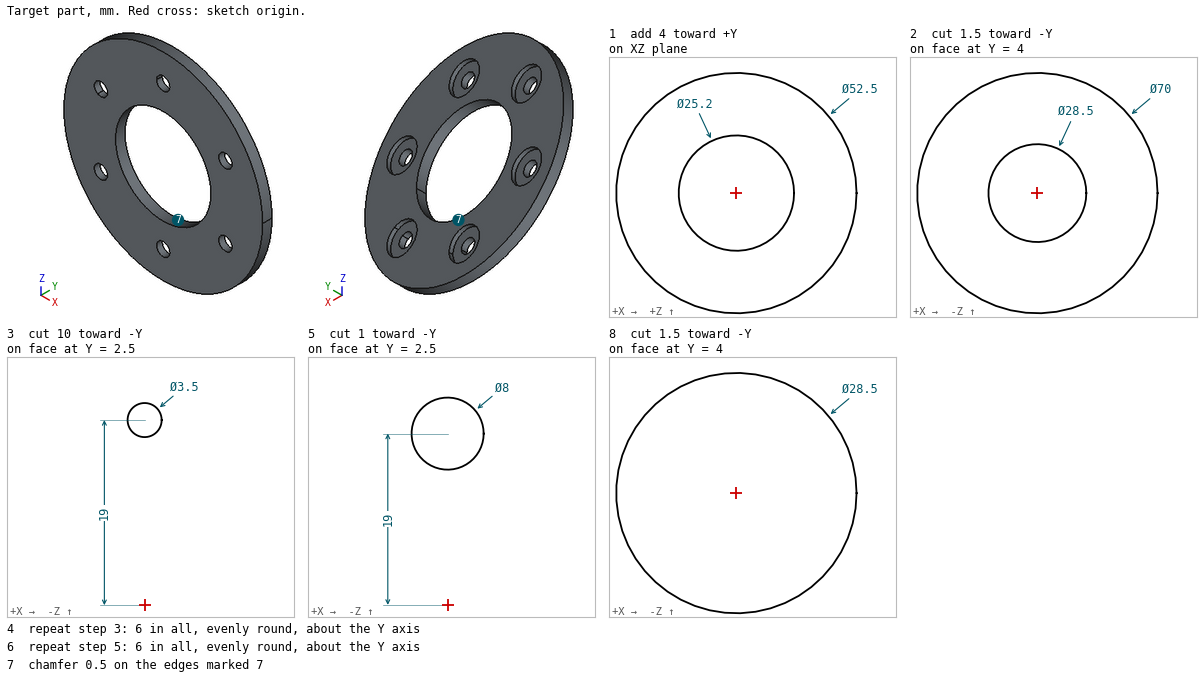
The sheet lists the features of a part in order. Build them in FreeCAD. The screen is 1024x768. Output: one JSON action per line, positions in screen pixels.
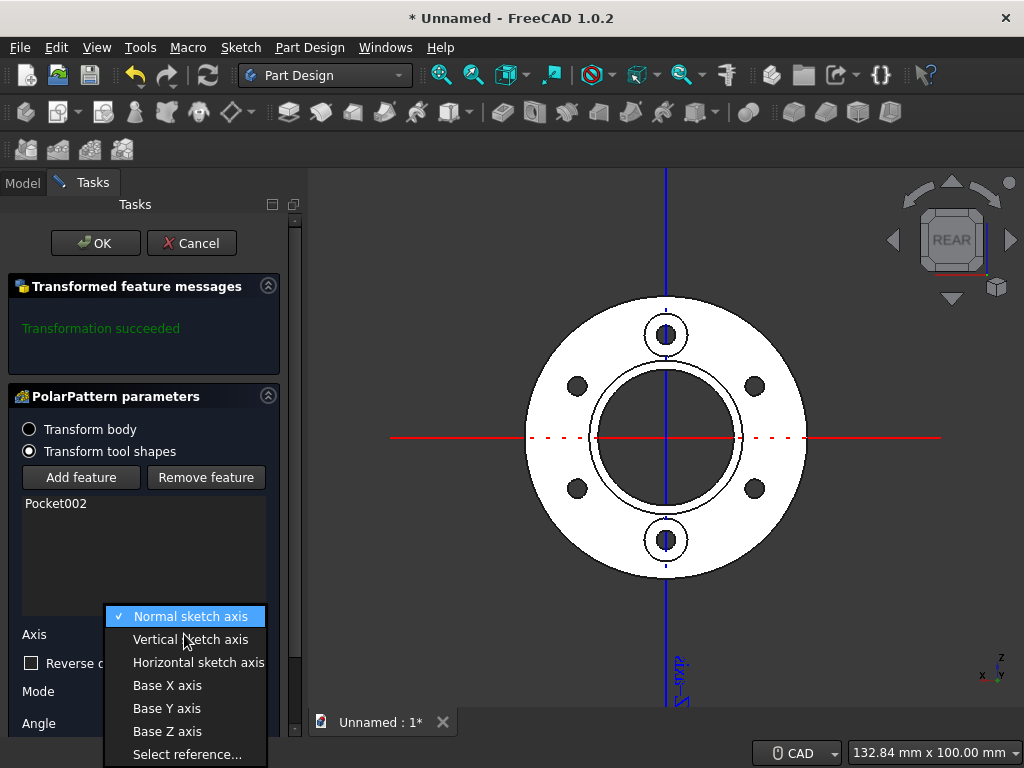
{"action": "left_click", "coordinate": [184, 708]}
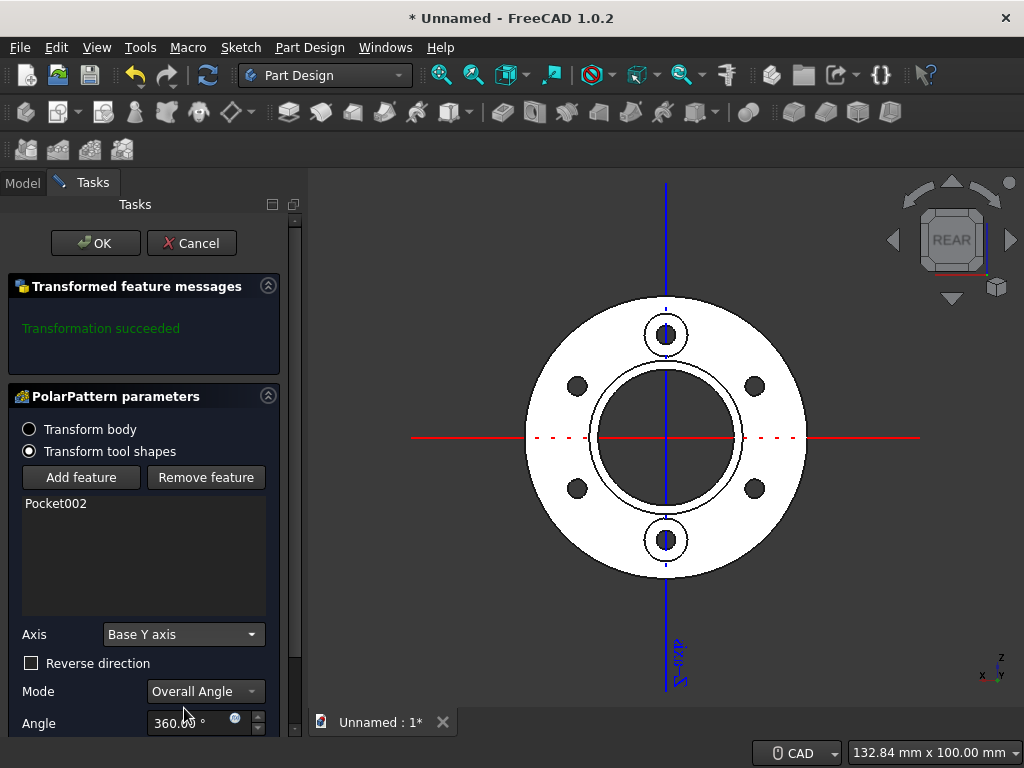
{"action": "scroll", "coordinate": [295, 475], "scroll_direction": "down", "scroll_amount": 2}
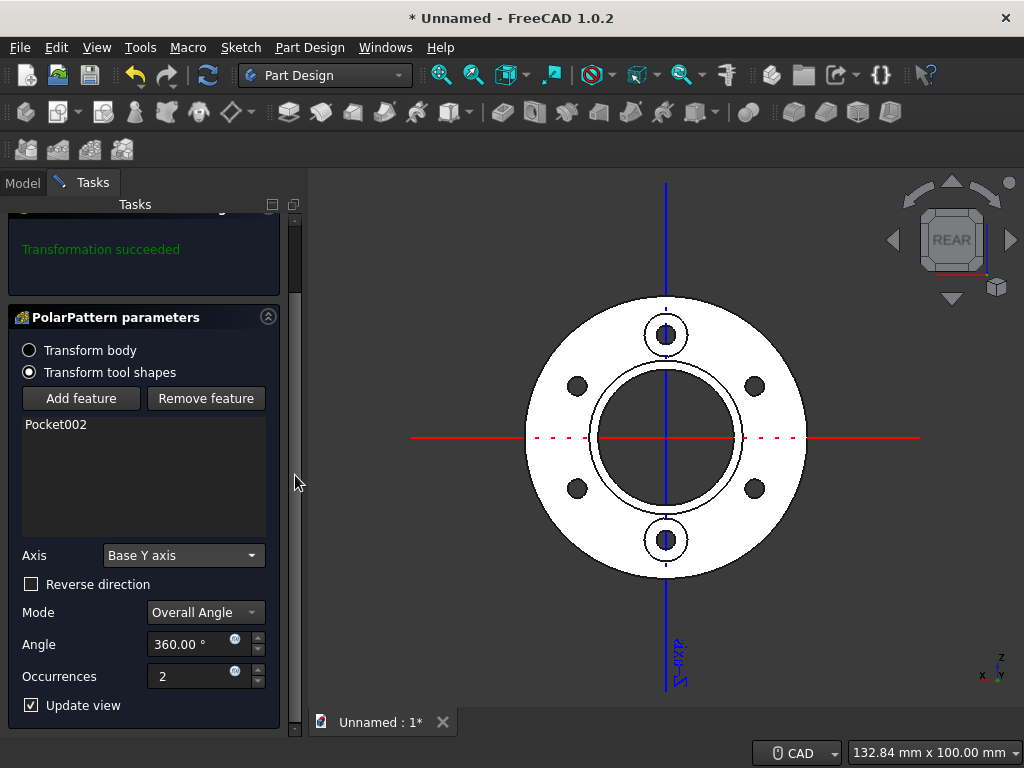
{"action": "triple_click", "coordinate": [198, 676]}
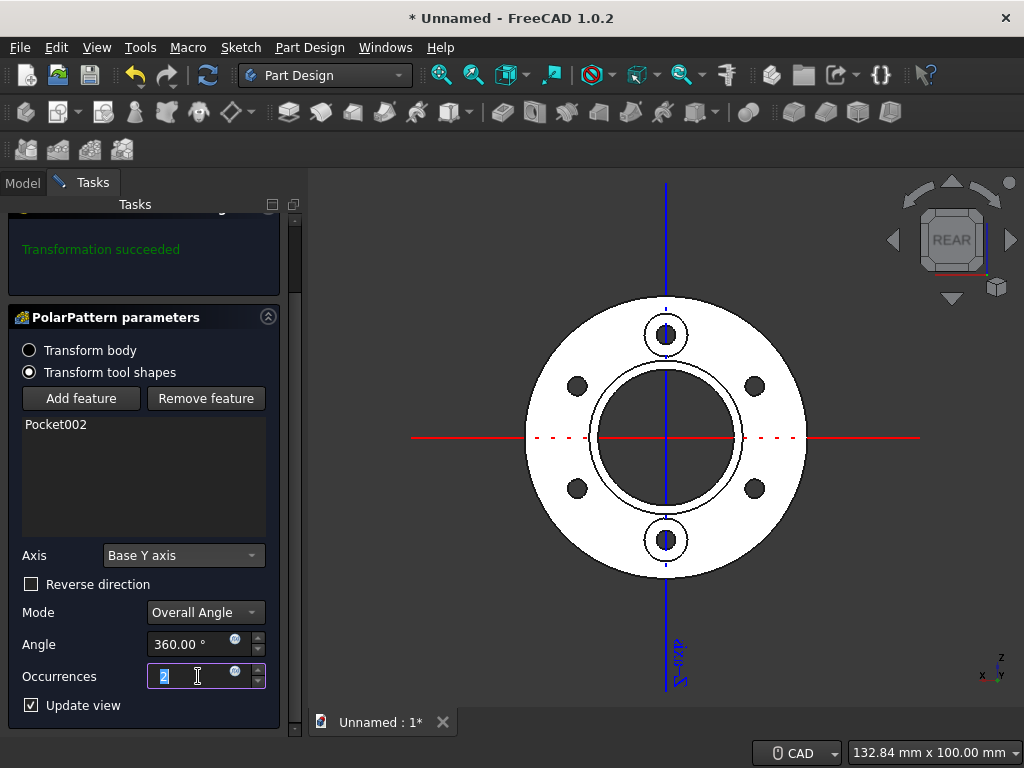
{"action": "type", "text": "6"}
{"action": "key", "text": "Tab"}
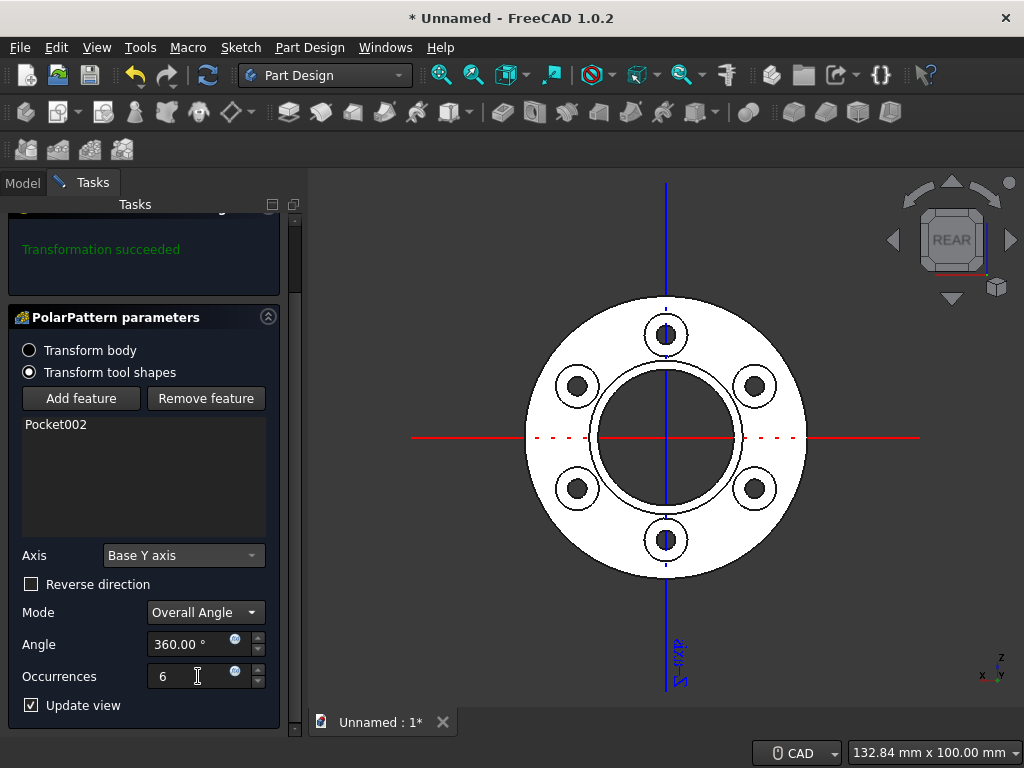
{"action": "scroll", "coordinate": [295, 475], "scroll_direction": "up", "scroll_amount": 3}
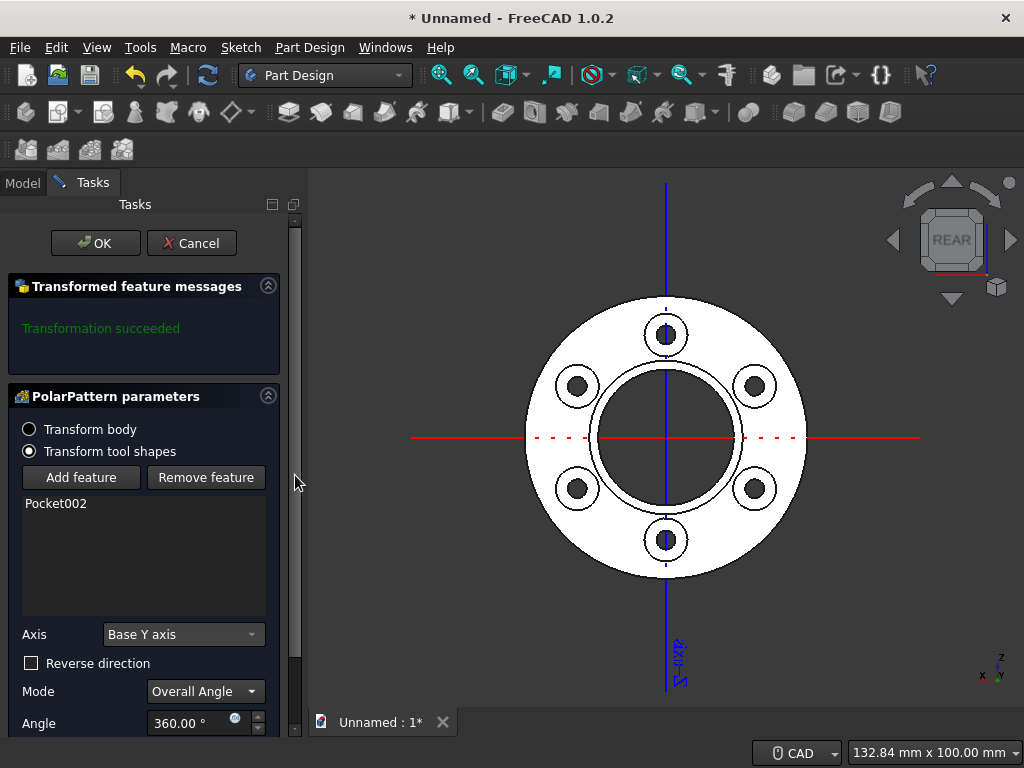
{"action": "left_click", "coordinate": [96, 243]}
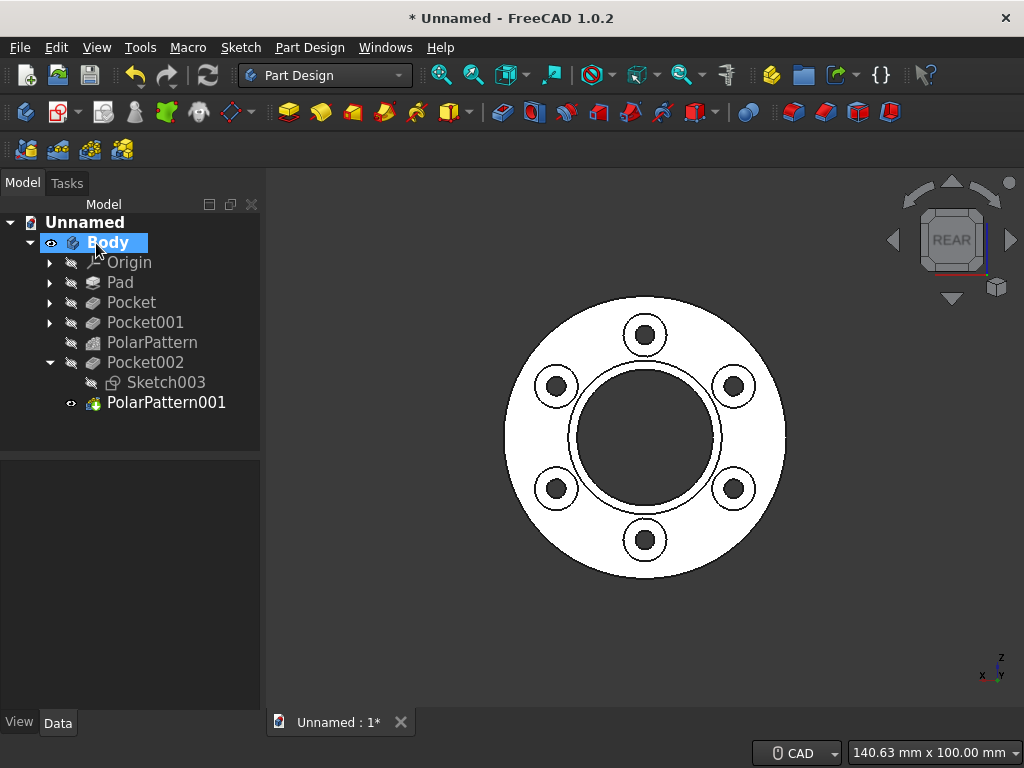
{"action": "left_click", "coordinate": [722, 436]}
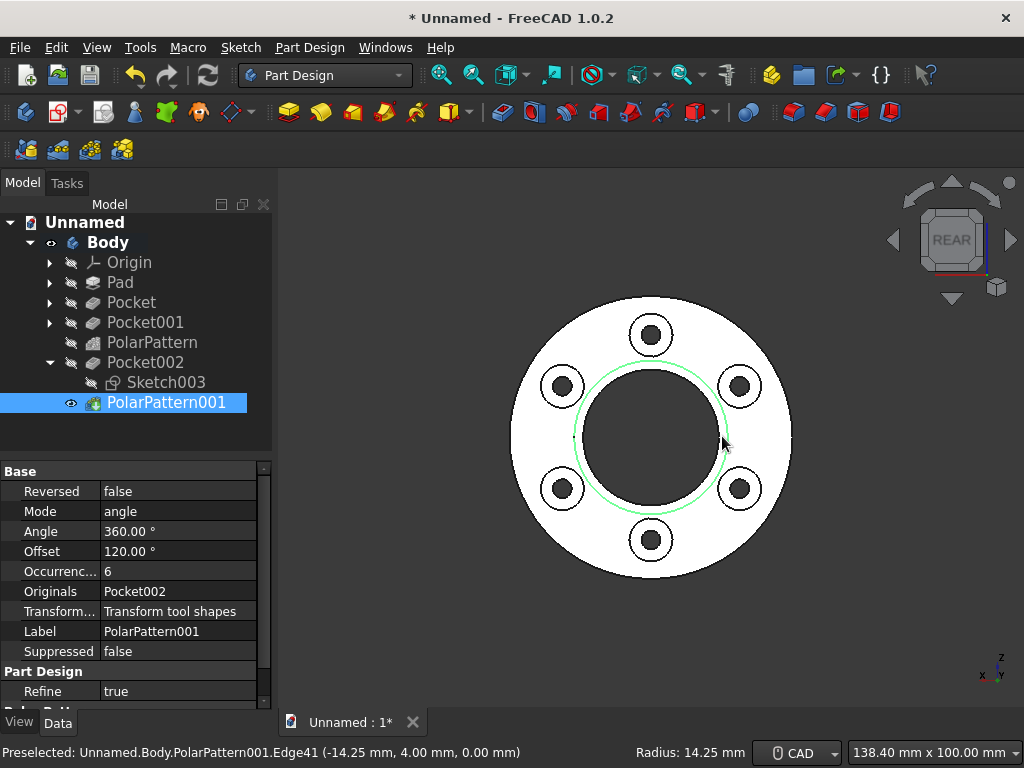
{"action": "left_click", "coordinate": [826, 112]}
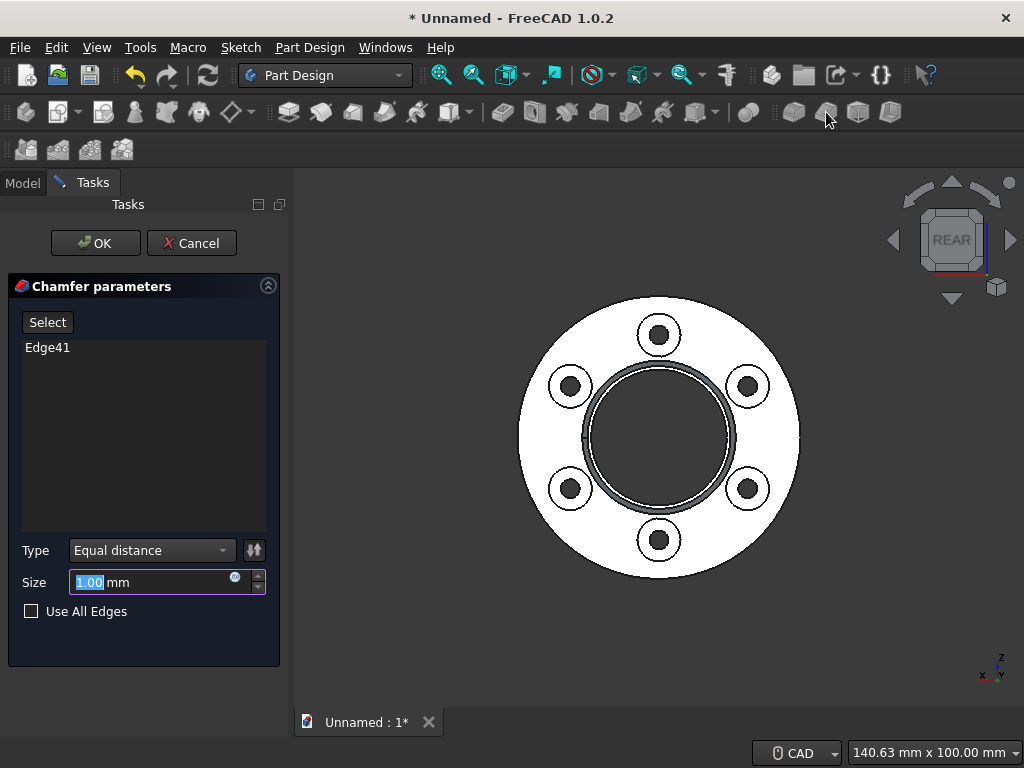
{"action": "type", "text": "0.5"}
{"action": "key", "text": "Tab"}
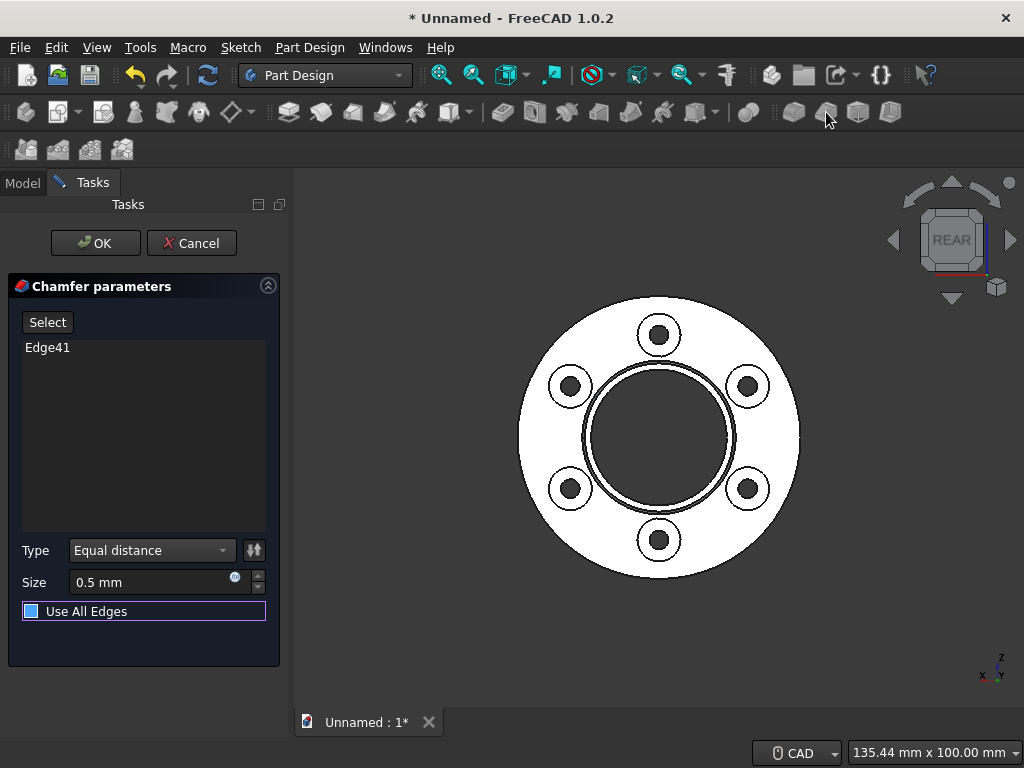
{"action": "left_click", "coordinate": [96, 243]}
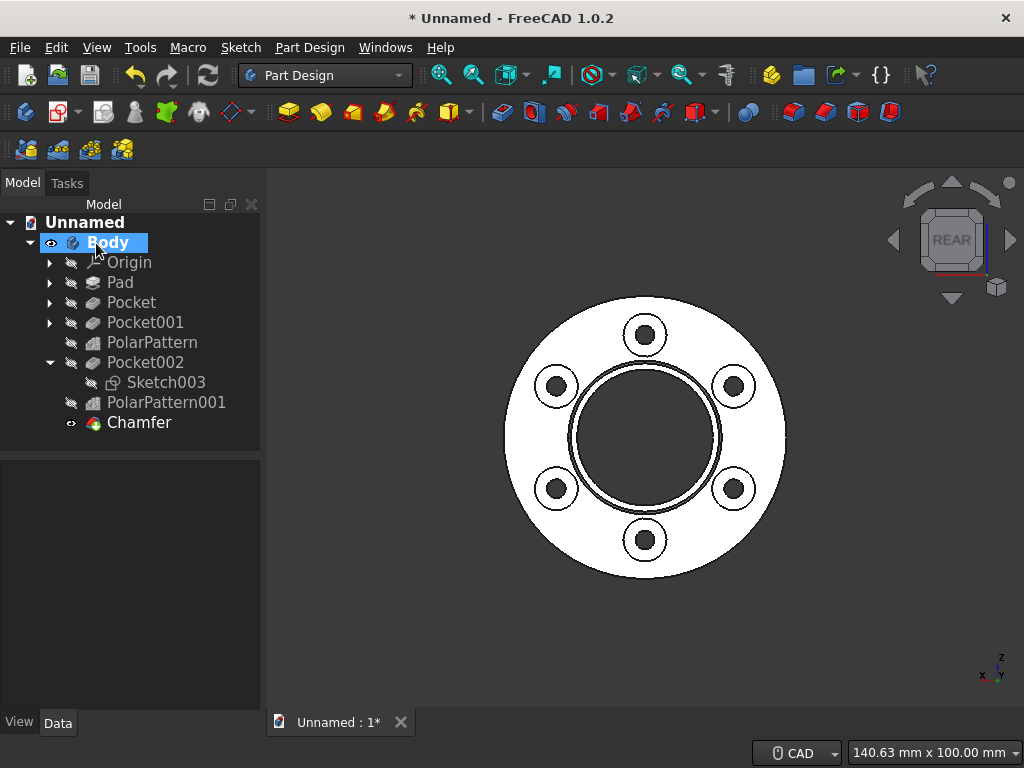
{"action": "scroll", "coordinate": [617, 370], "scroll_direction": "up", "scroll_amount": 9}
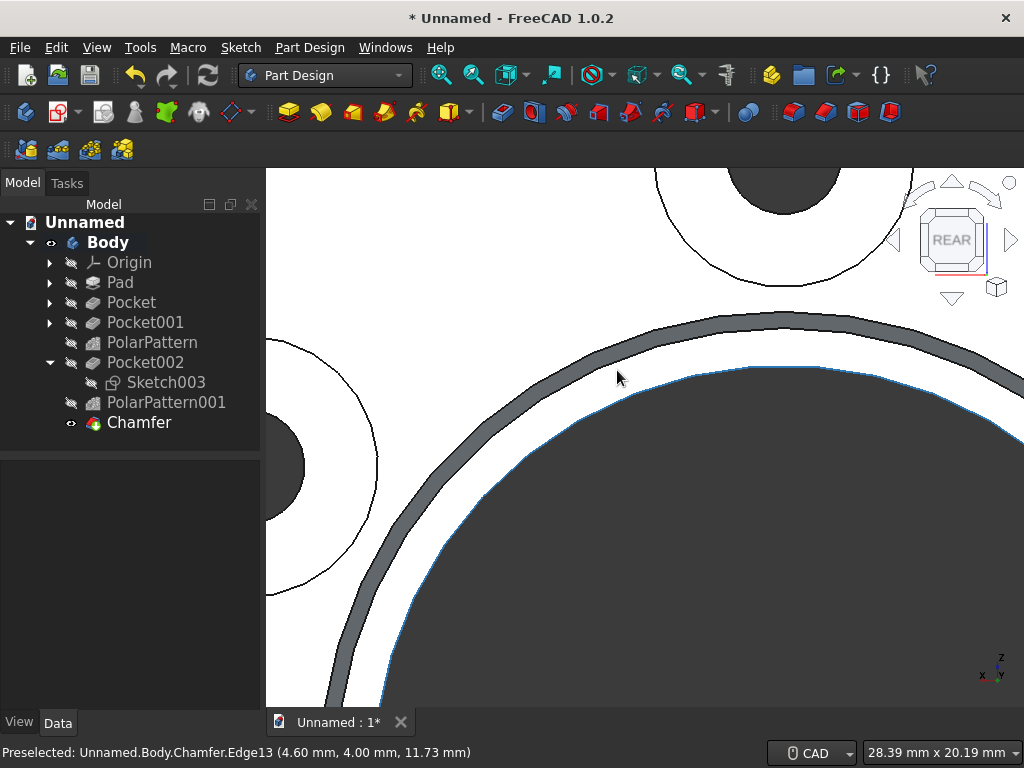
{"action": "left_click", "coordinate": [612, 375]}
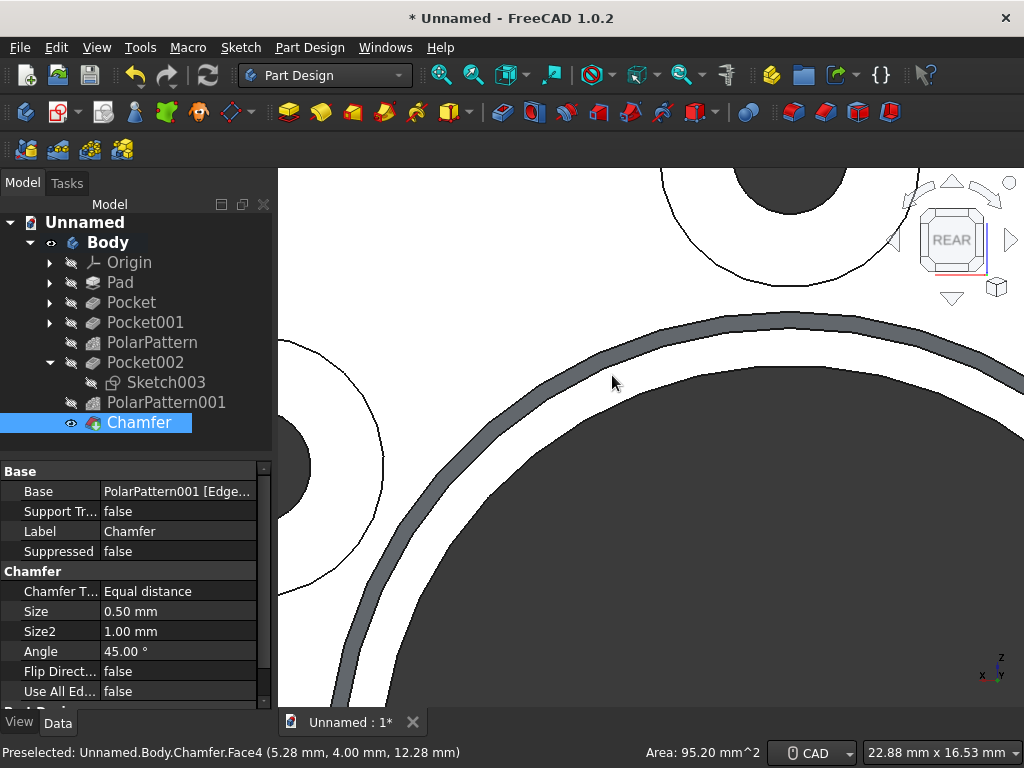
{"action": "left_click", "coordinate": [58, 112]}